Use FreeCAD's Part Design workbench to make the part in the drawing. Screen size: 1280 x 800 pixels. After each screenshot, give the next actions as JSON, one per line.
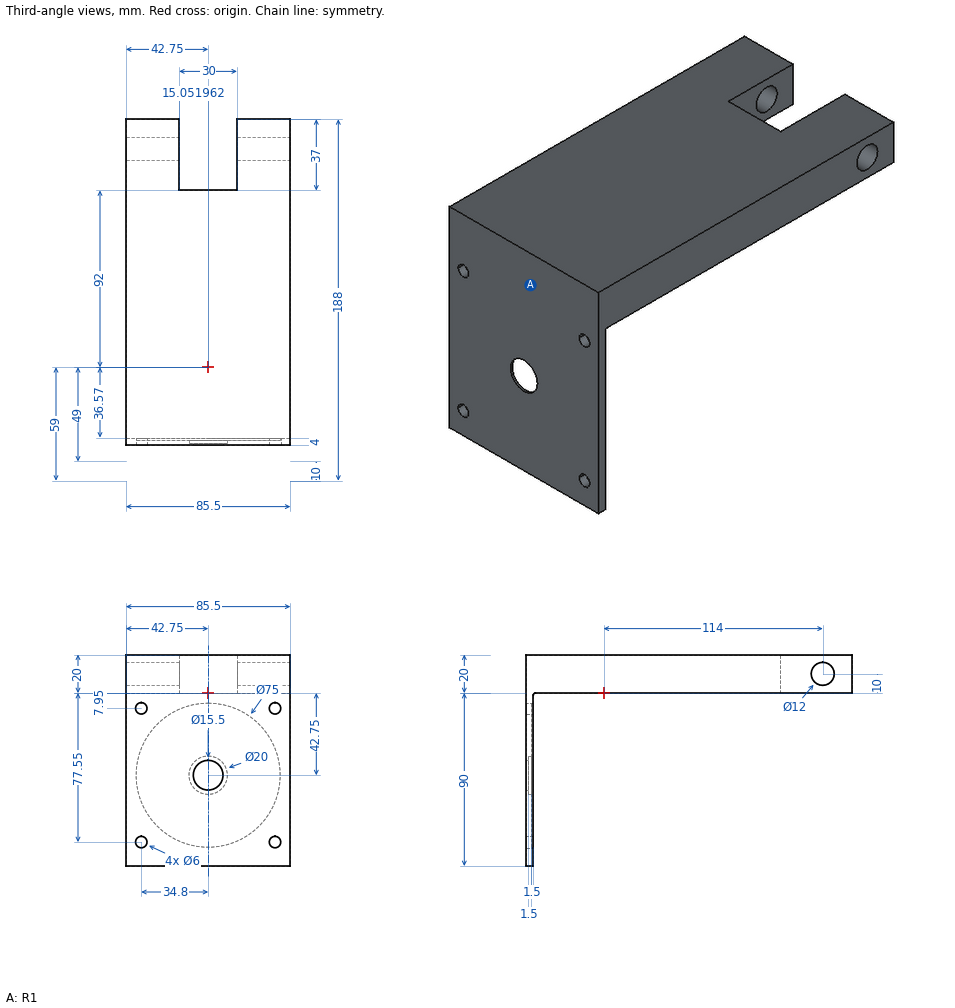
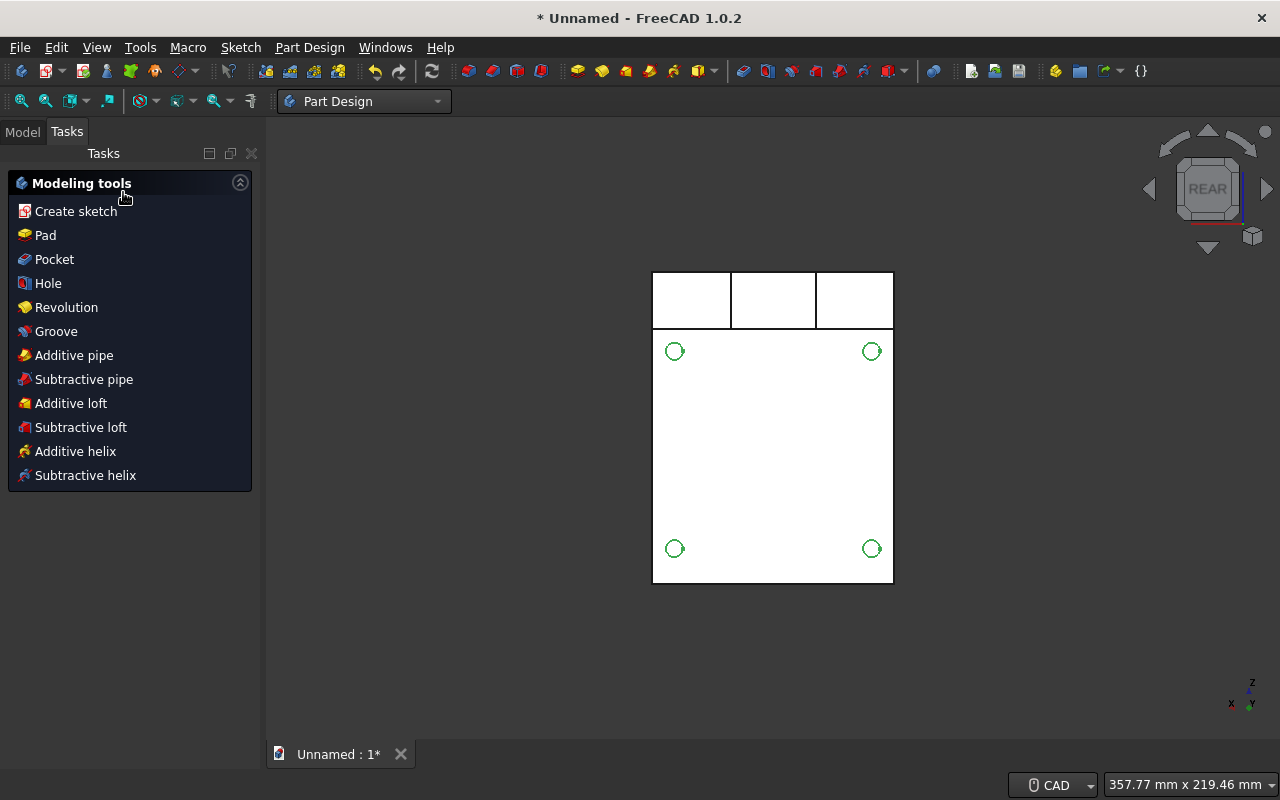
{"action": "left_click", "coordinate": [744, 72]}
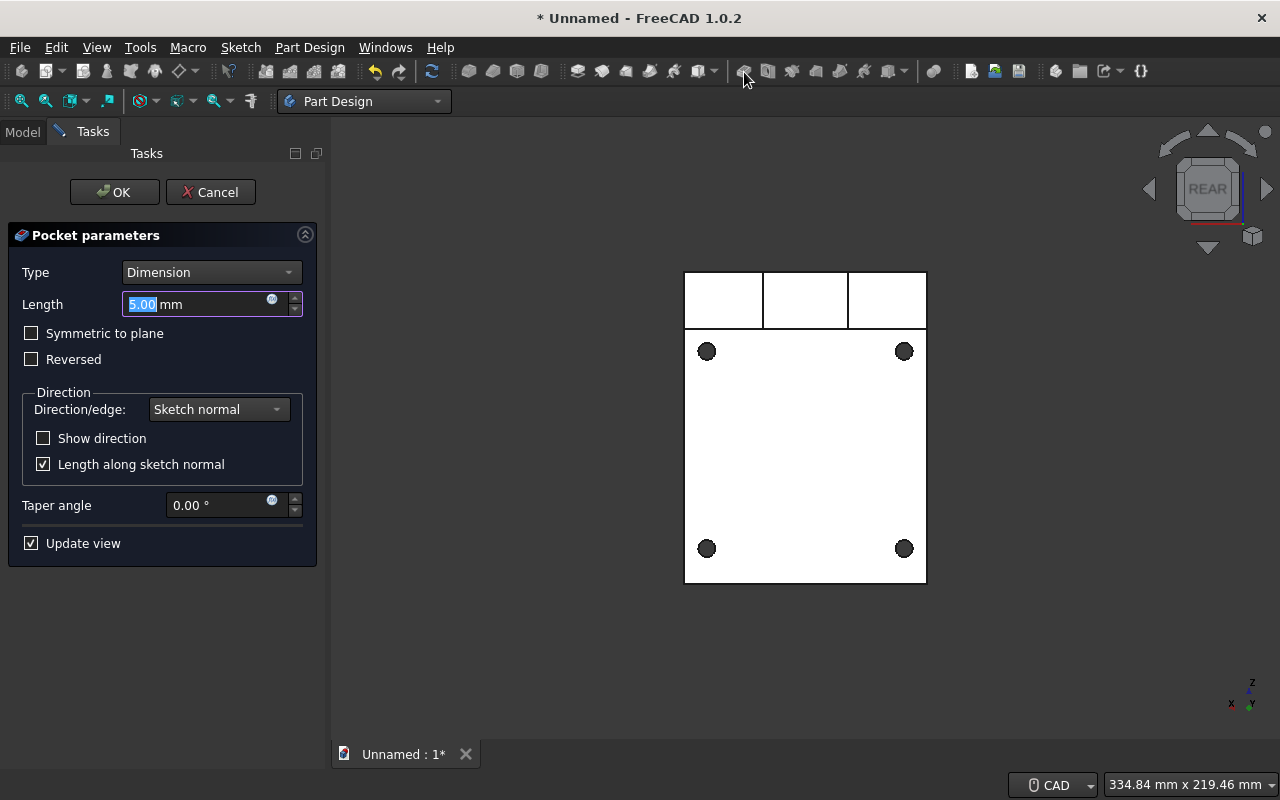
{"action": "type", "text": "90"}
{"action": "key", "text": "Tab"}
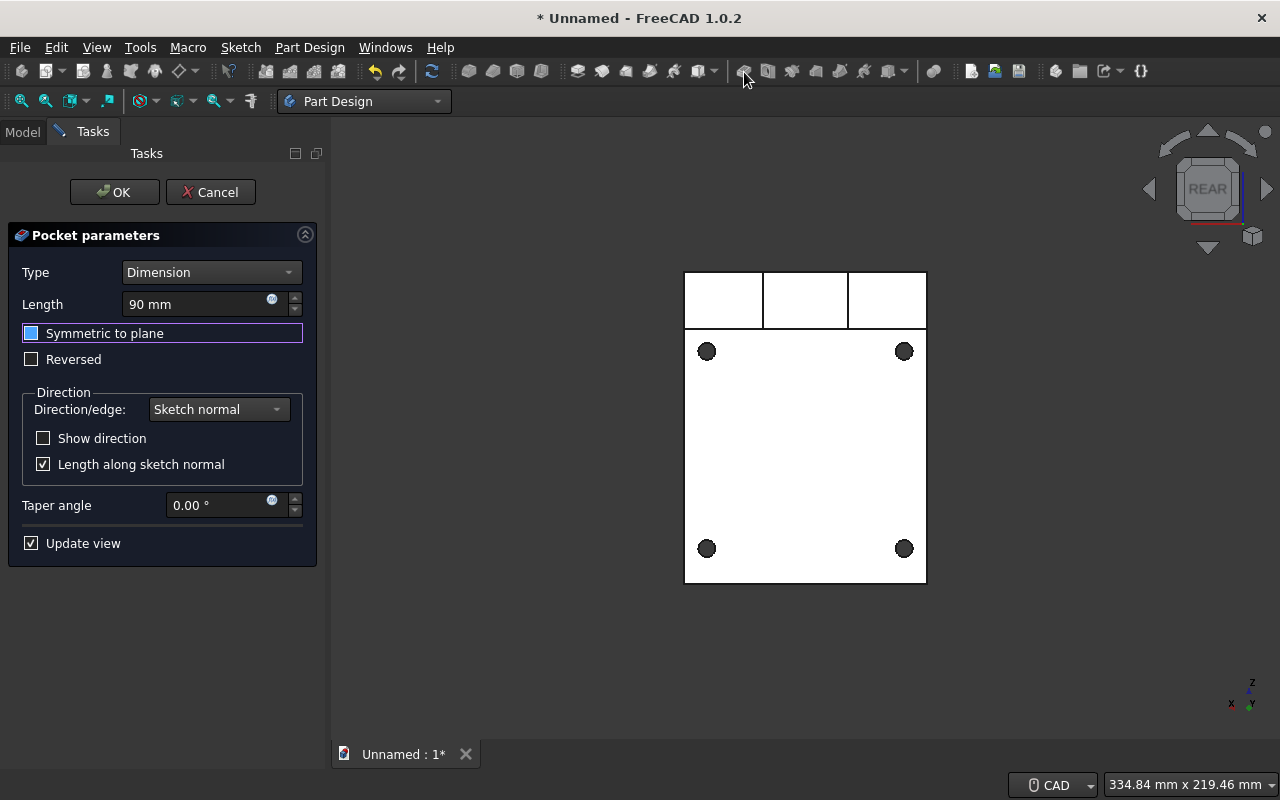
{"action": "left_click", "coordinate": [115, 192]}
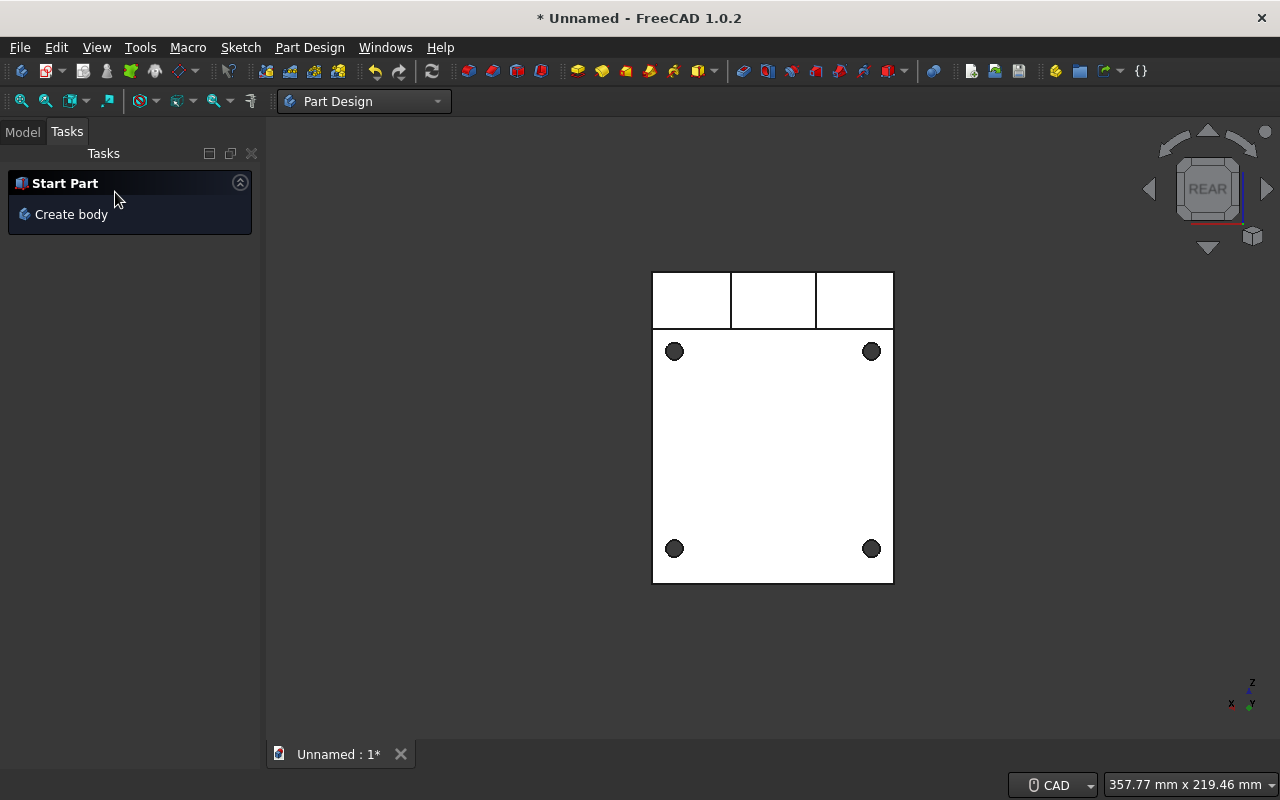
{"action": "key", "text": "0"}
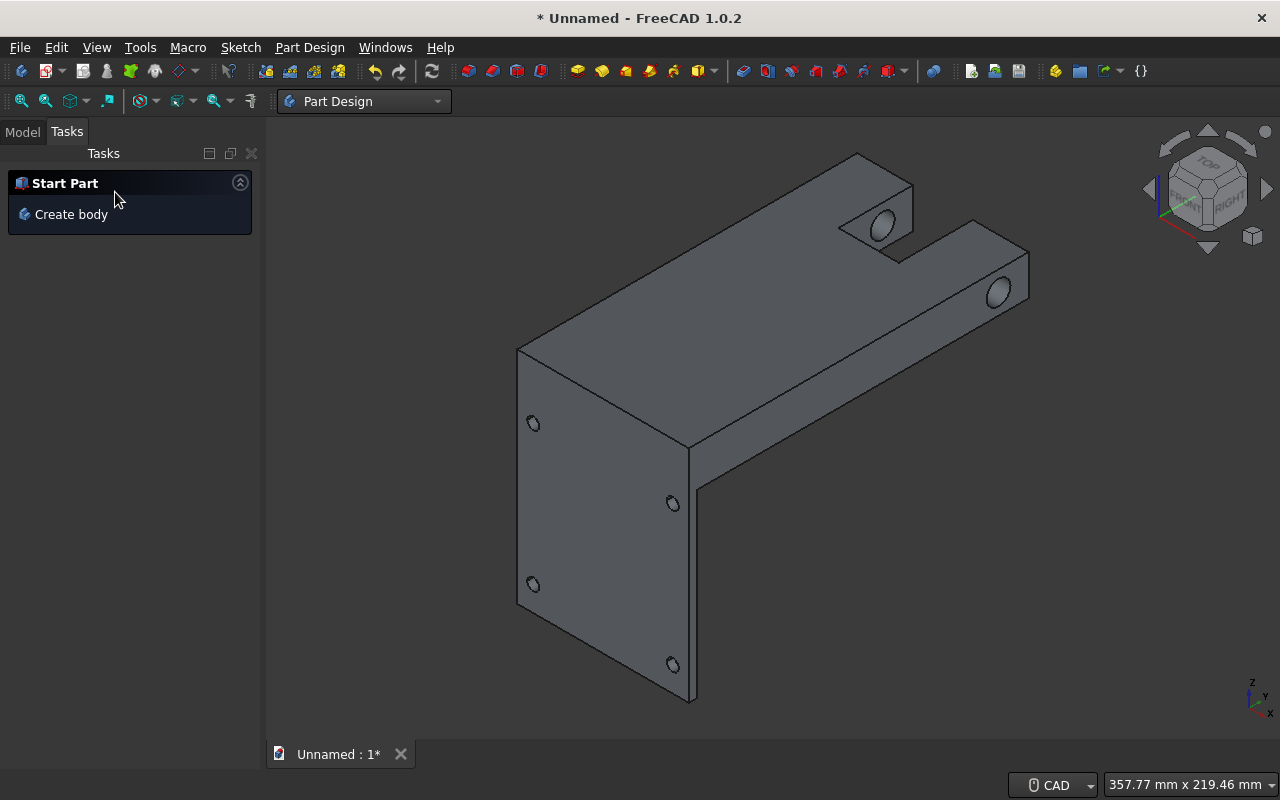
{"action": "key", "text": "2"}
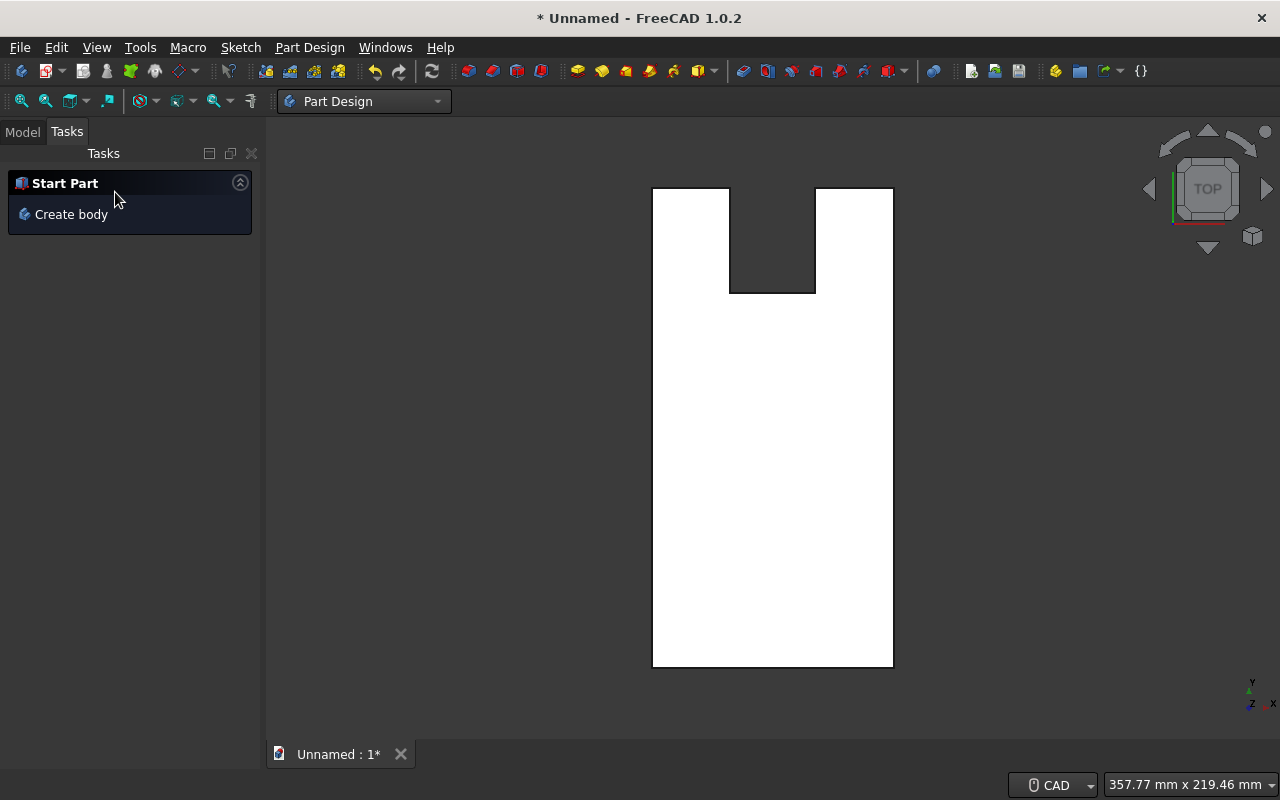
{"action": "key", "text": "1"}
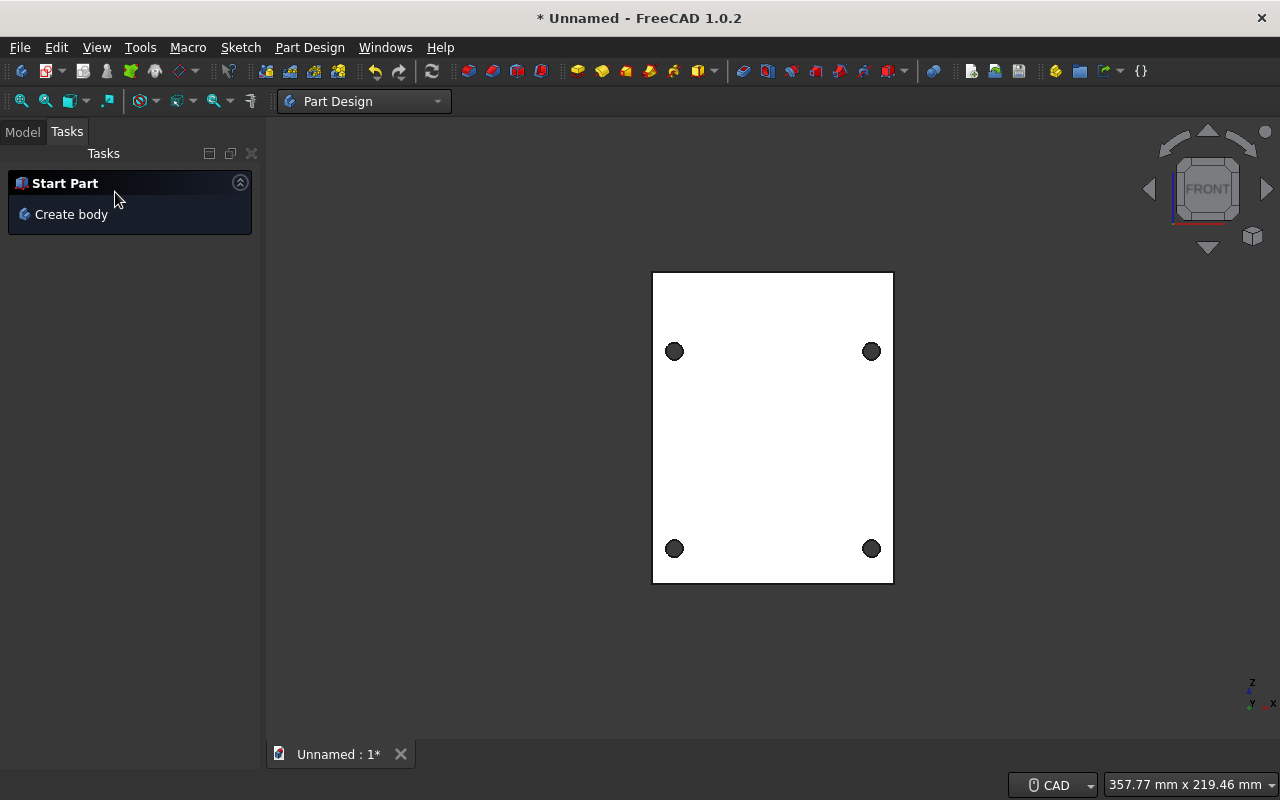
{"action": "key", "text": "3"}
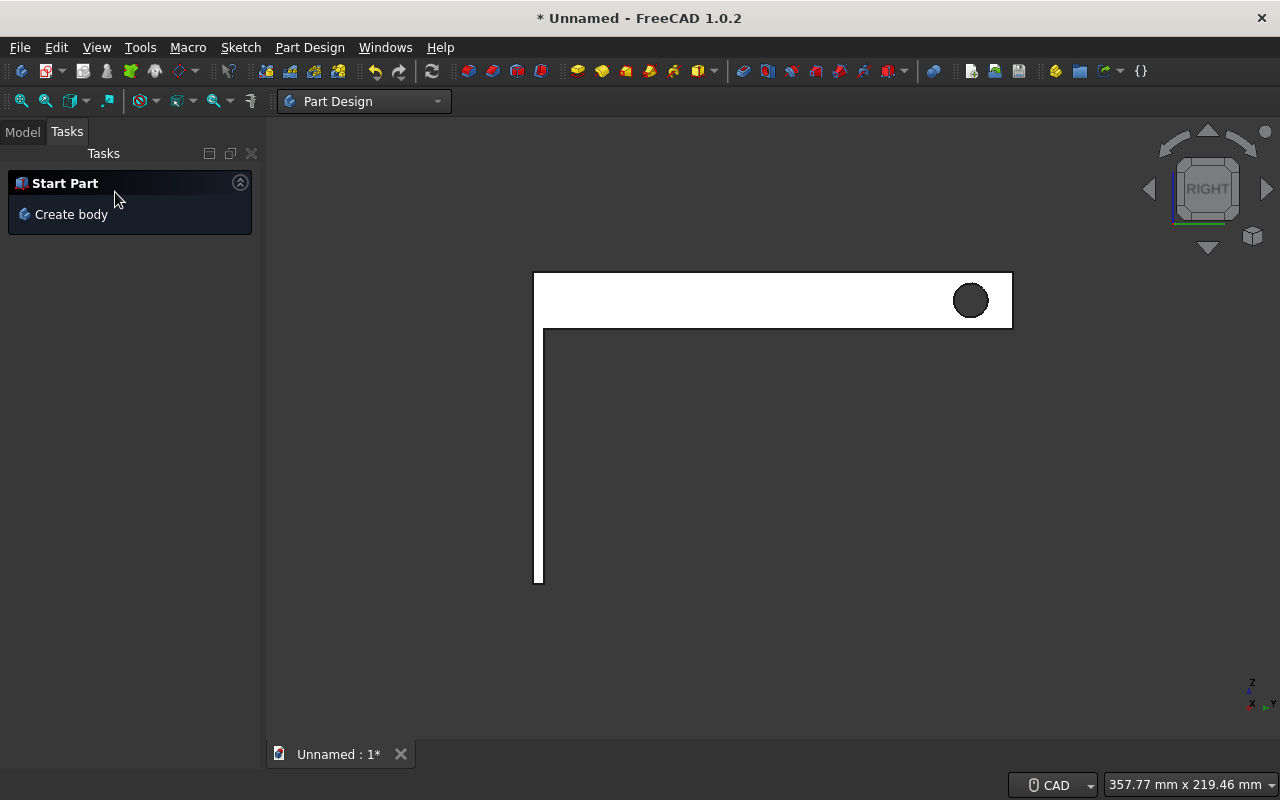
{"action": "key", "text": "5"}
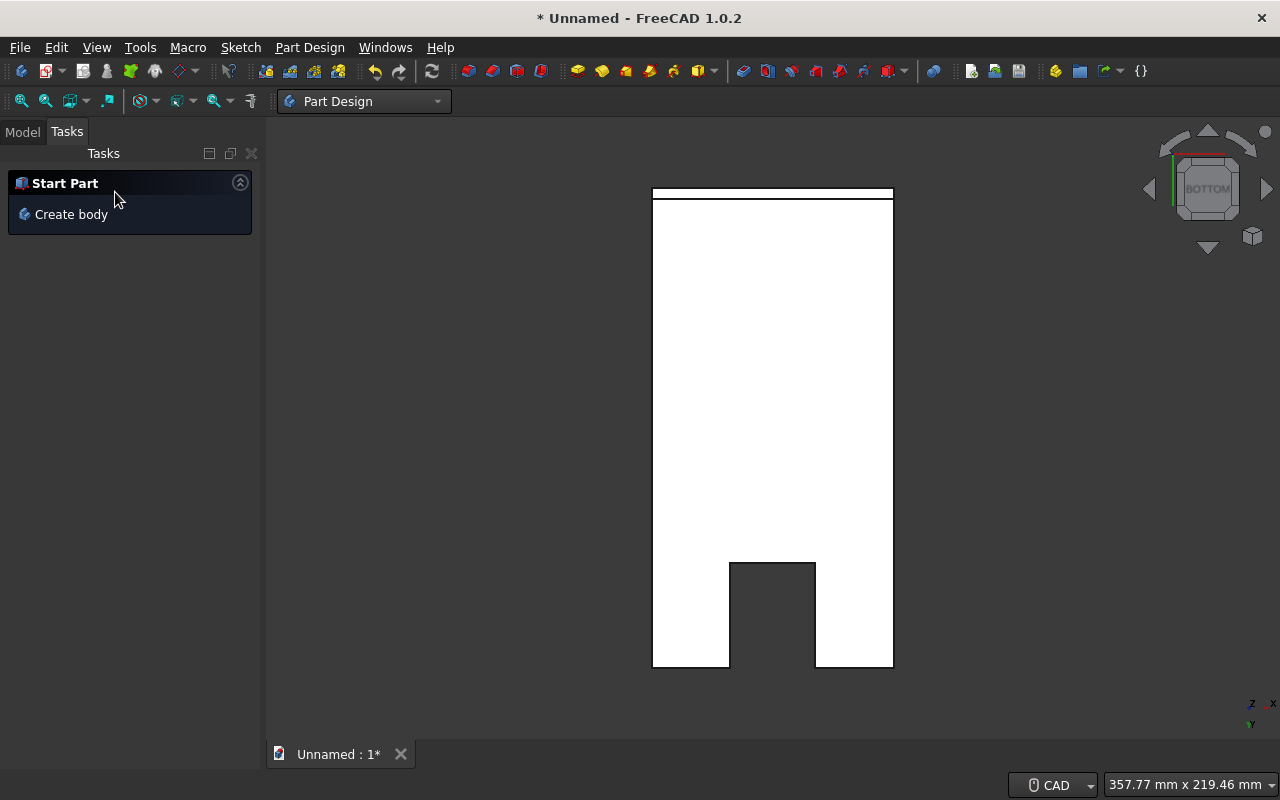
{"action": "key", "text": "4"}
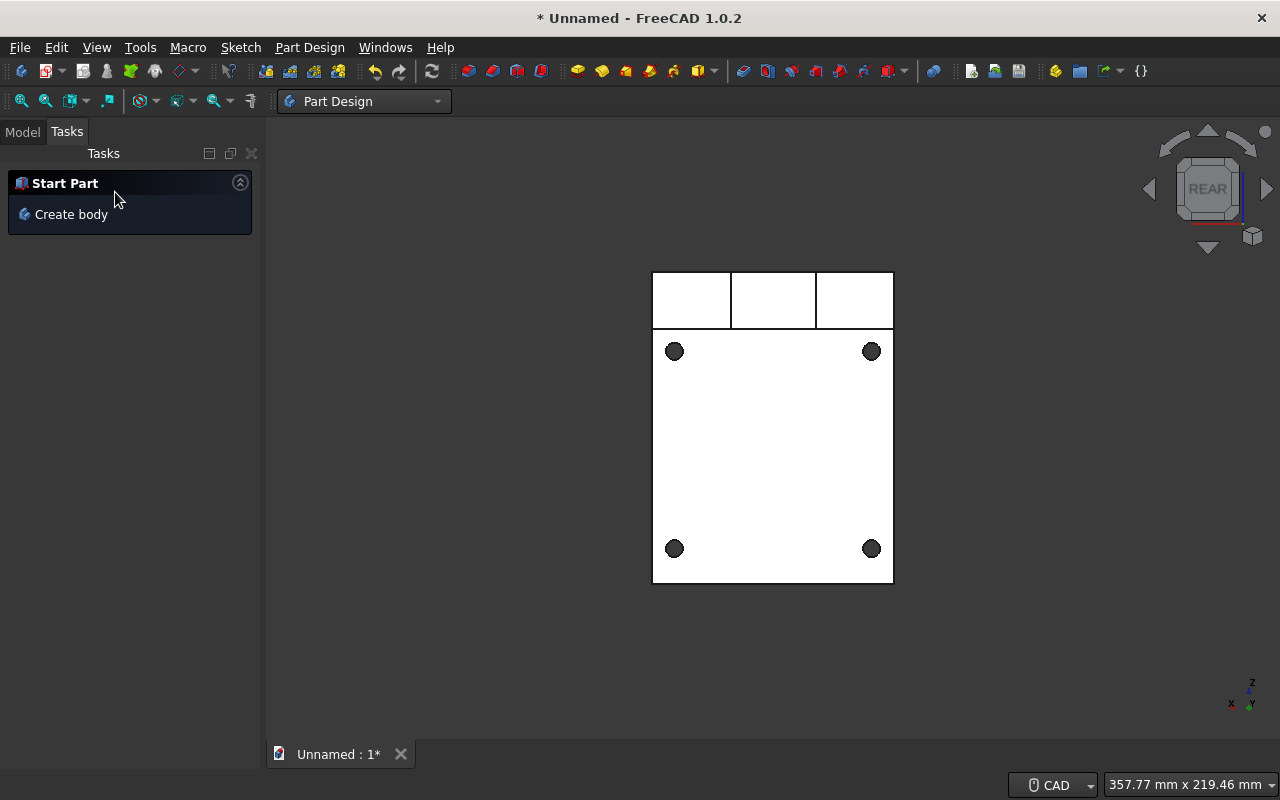
{"action": "key", "text": "6"}